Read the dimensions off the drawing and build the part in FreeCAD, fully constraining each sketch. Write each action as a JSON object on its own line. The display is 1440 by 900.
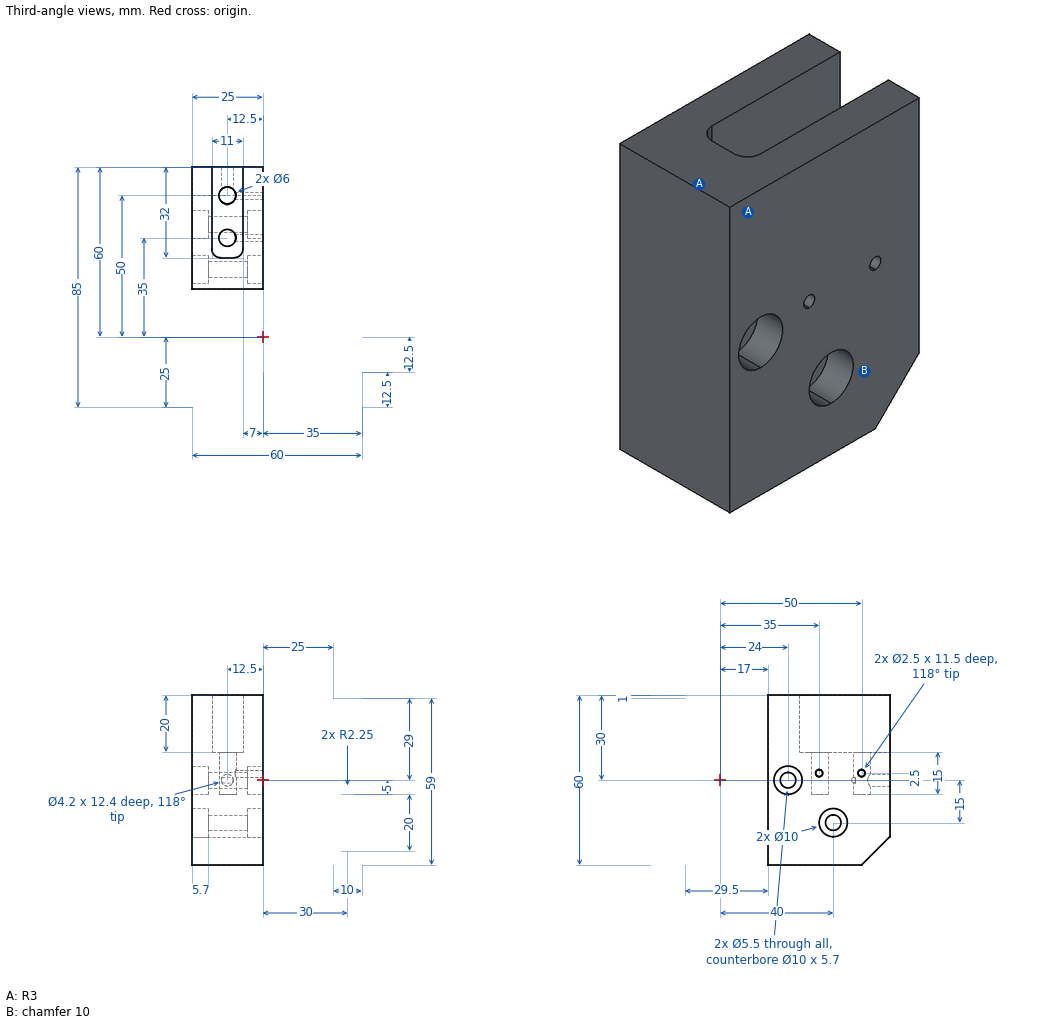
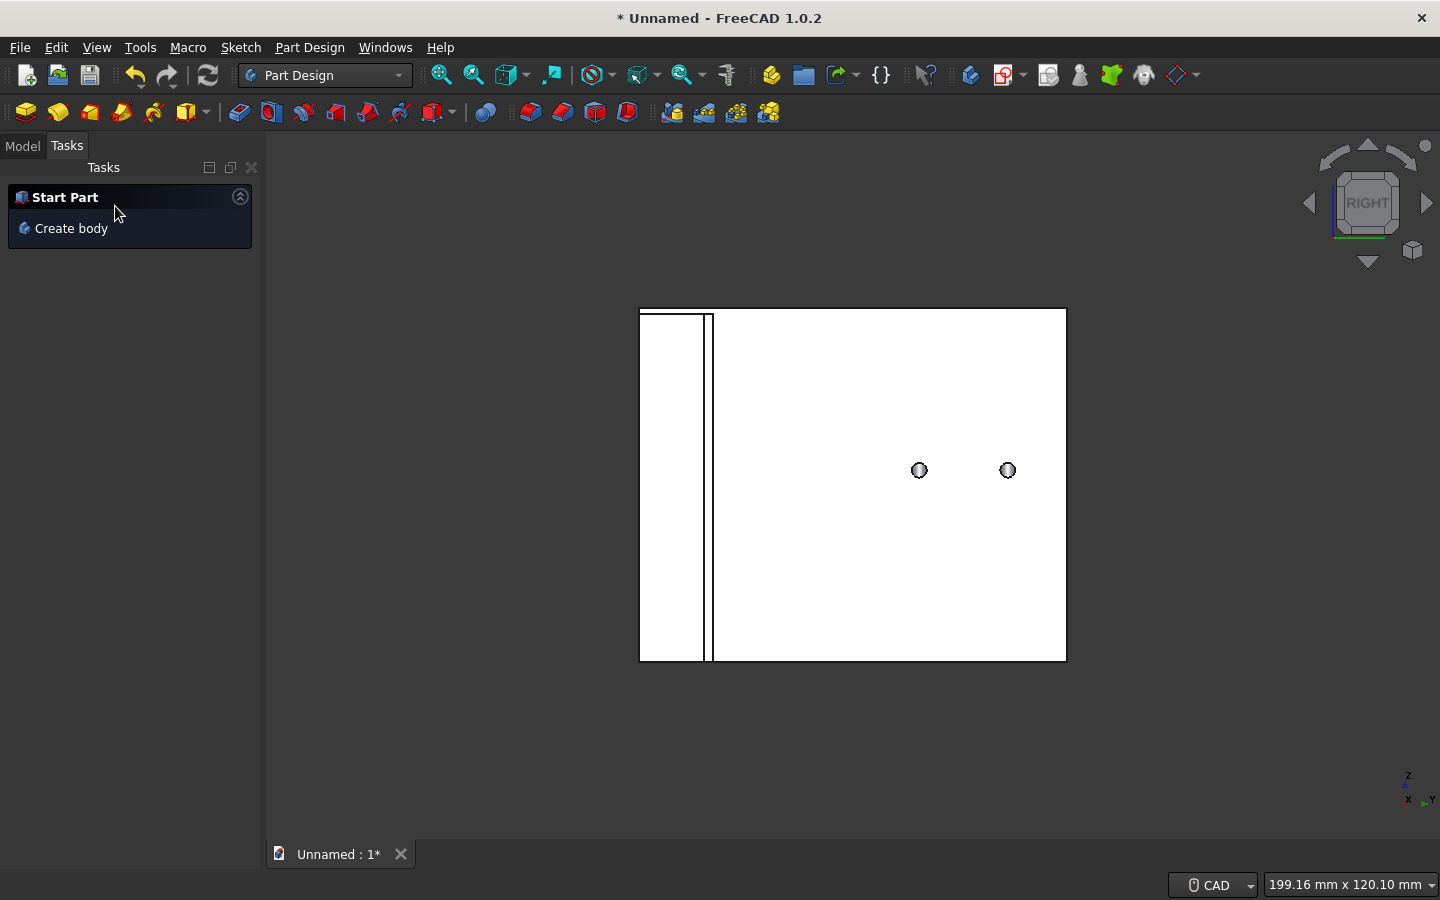
{"action": "key", "text": "5"}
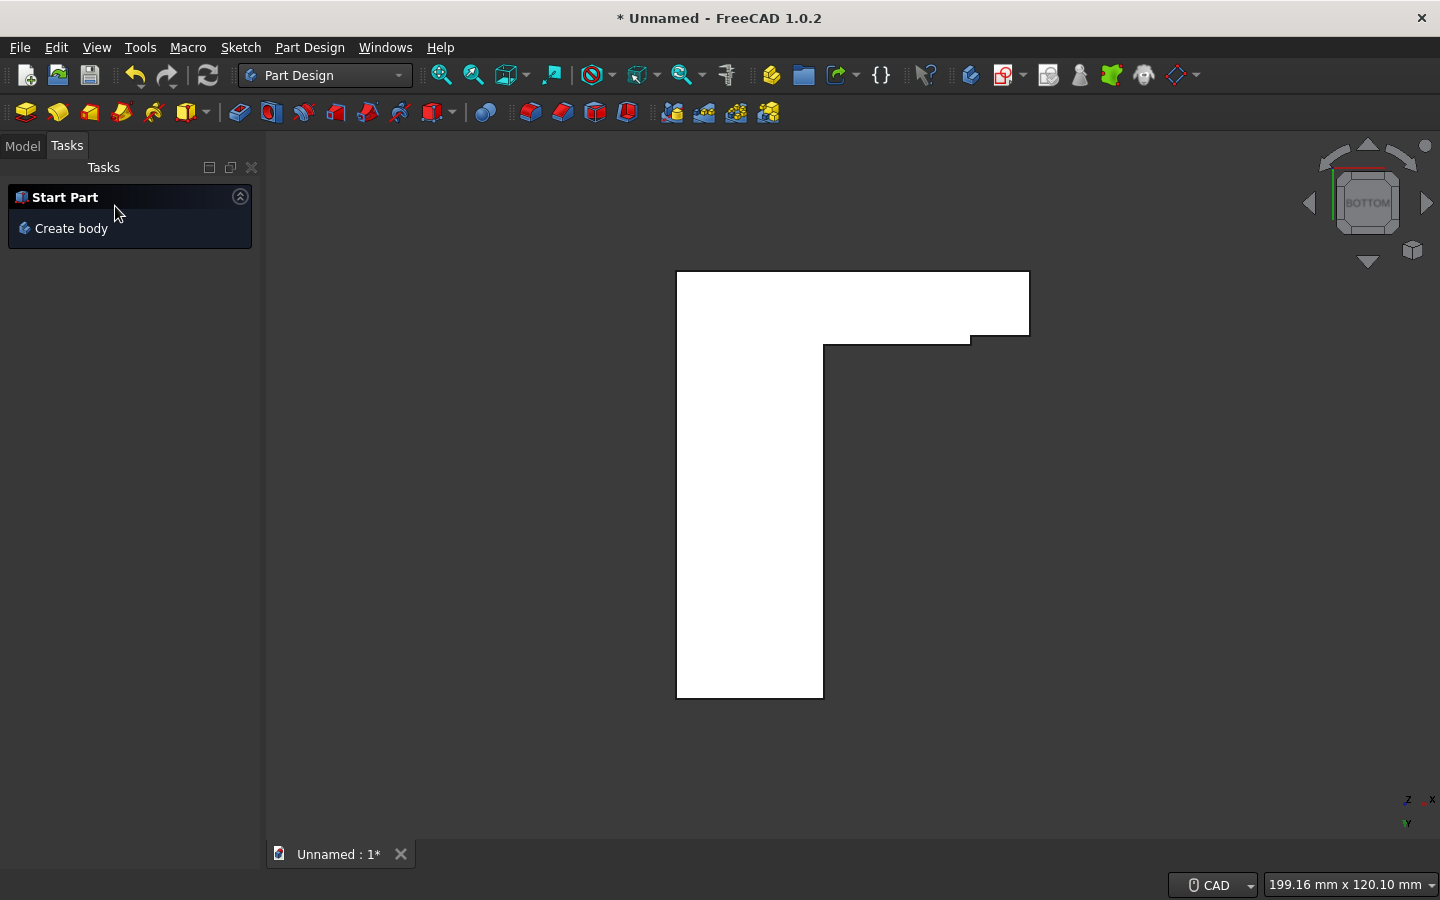
{"action": "left_click", "coordinate": [750, 698]}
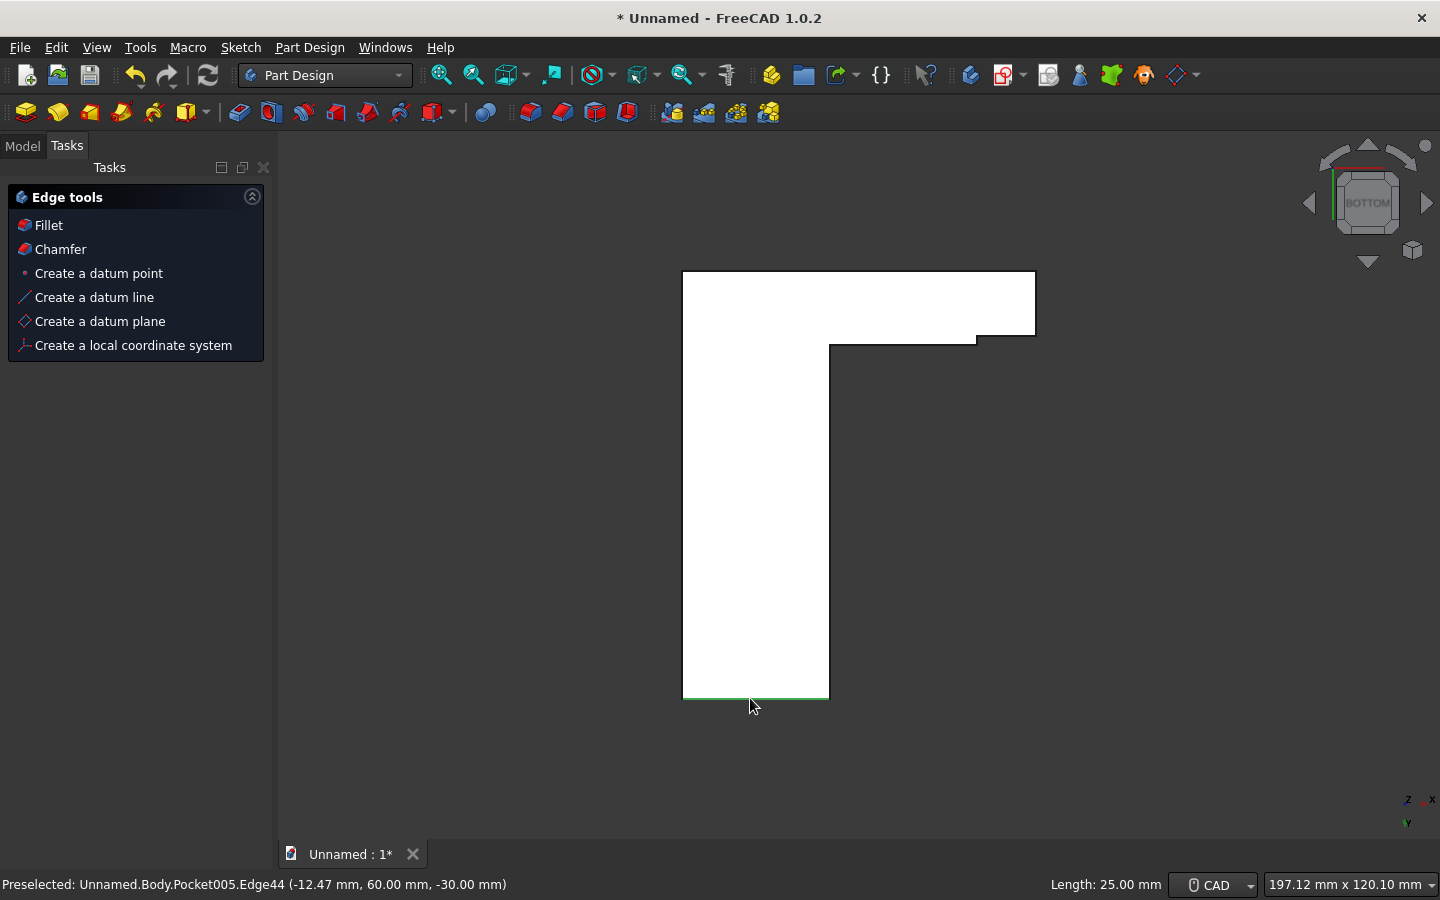
{"action": "left_click", "coordinate": [564, 112]}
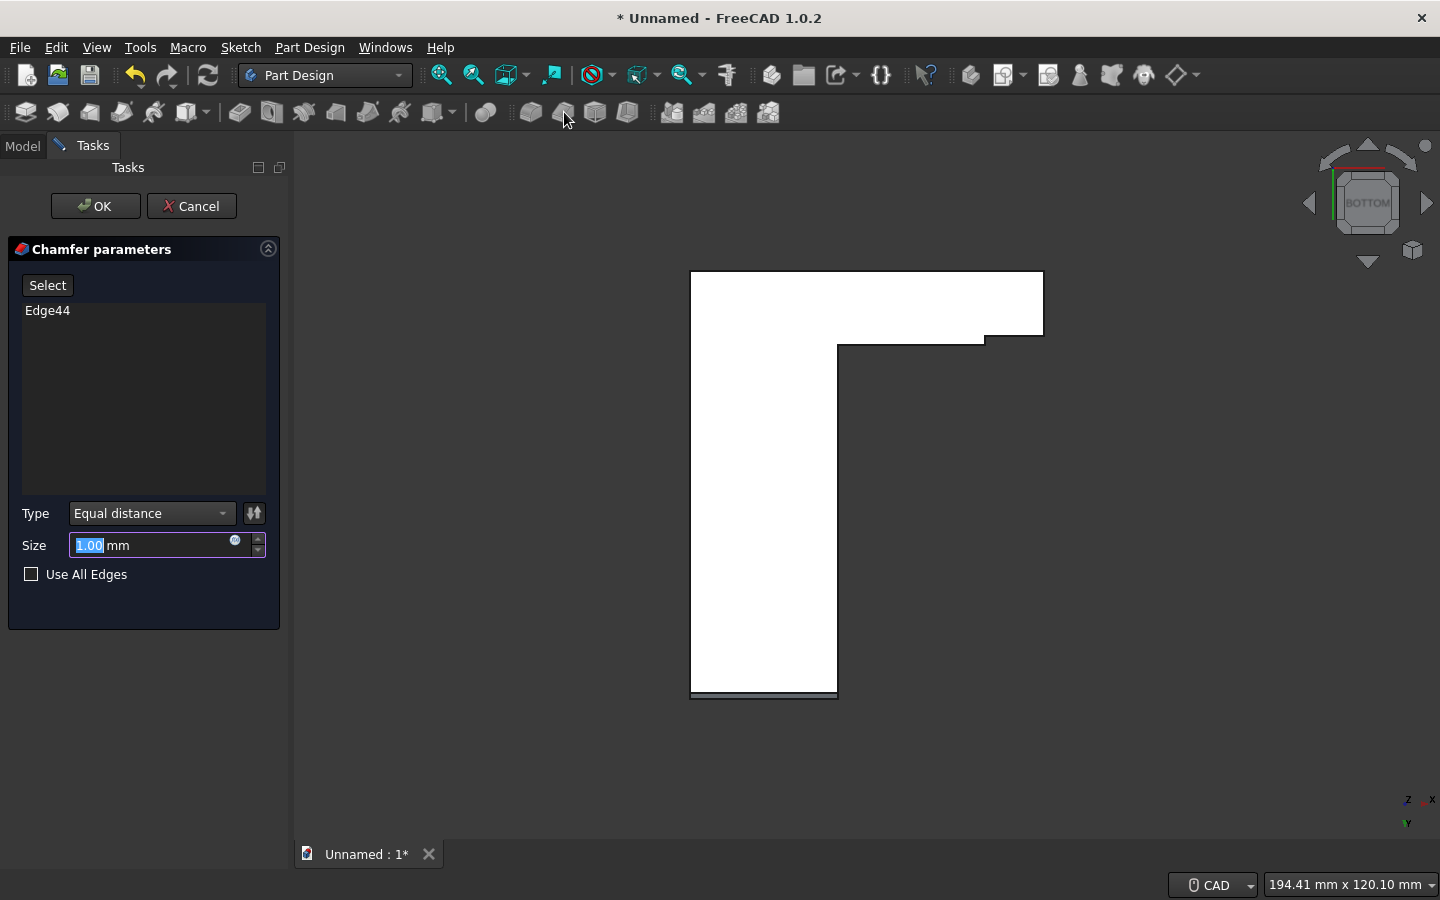
{"action": "type", "text": "10"}
{"action": "key", "text": "Tab"}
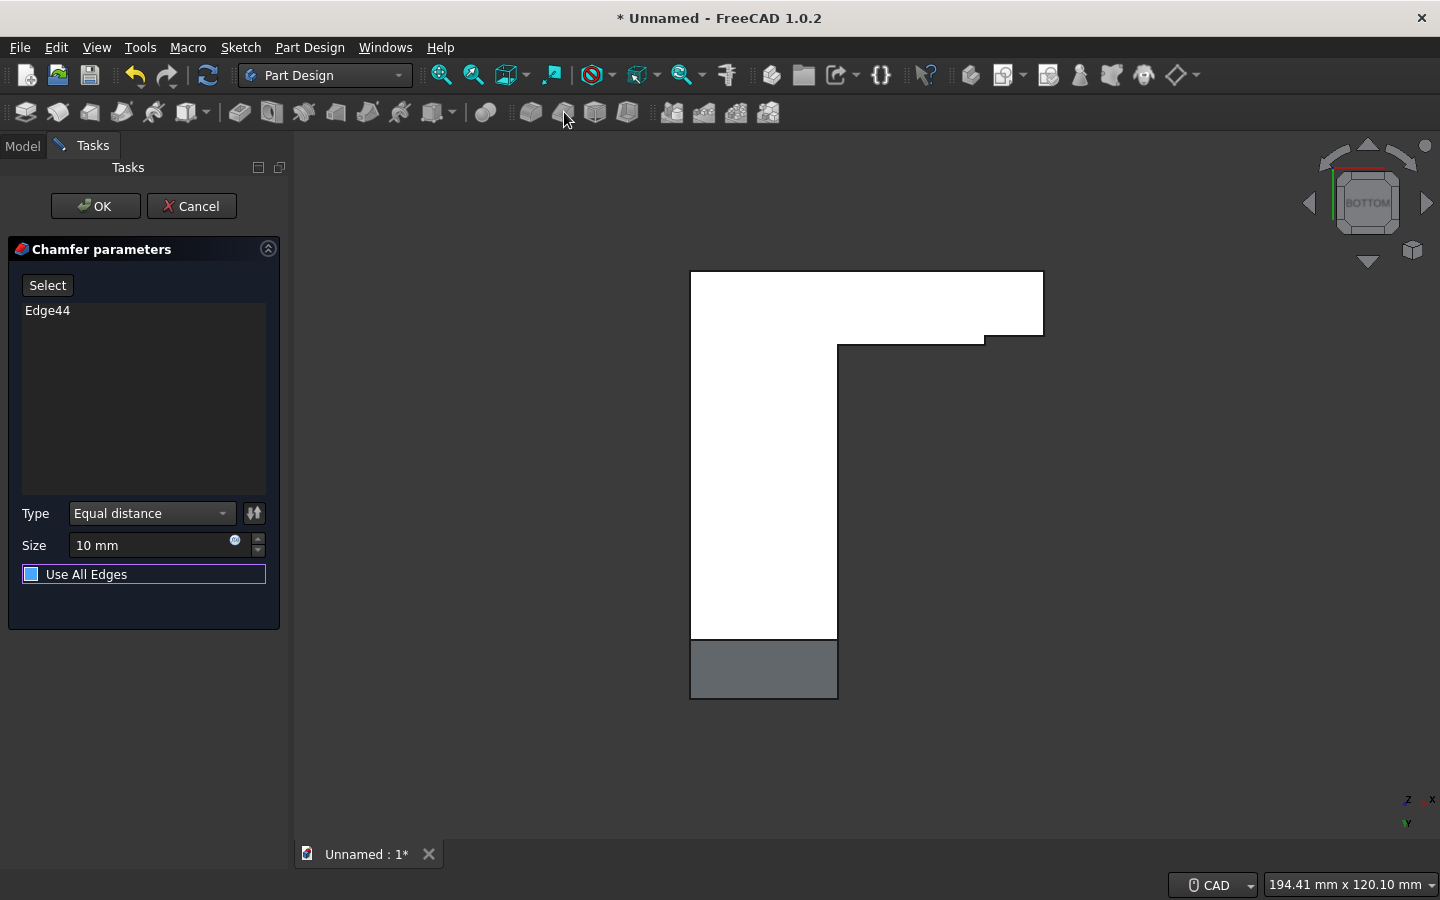
{"action": "left_click", "coordinate": [96, 206]}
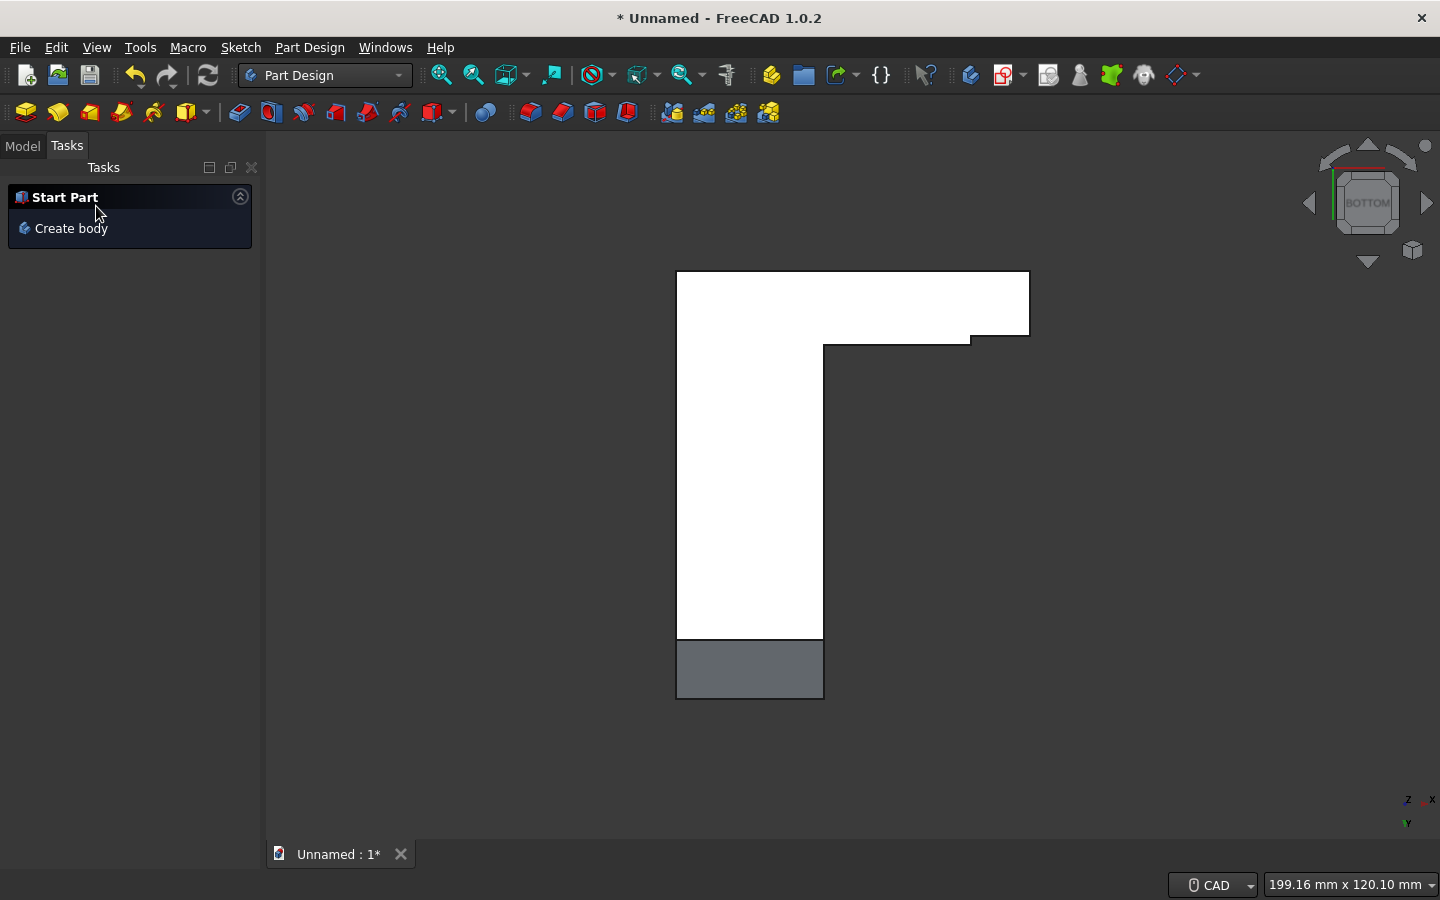
{"action": "key", "text": "0"}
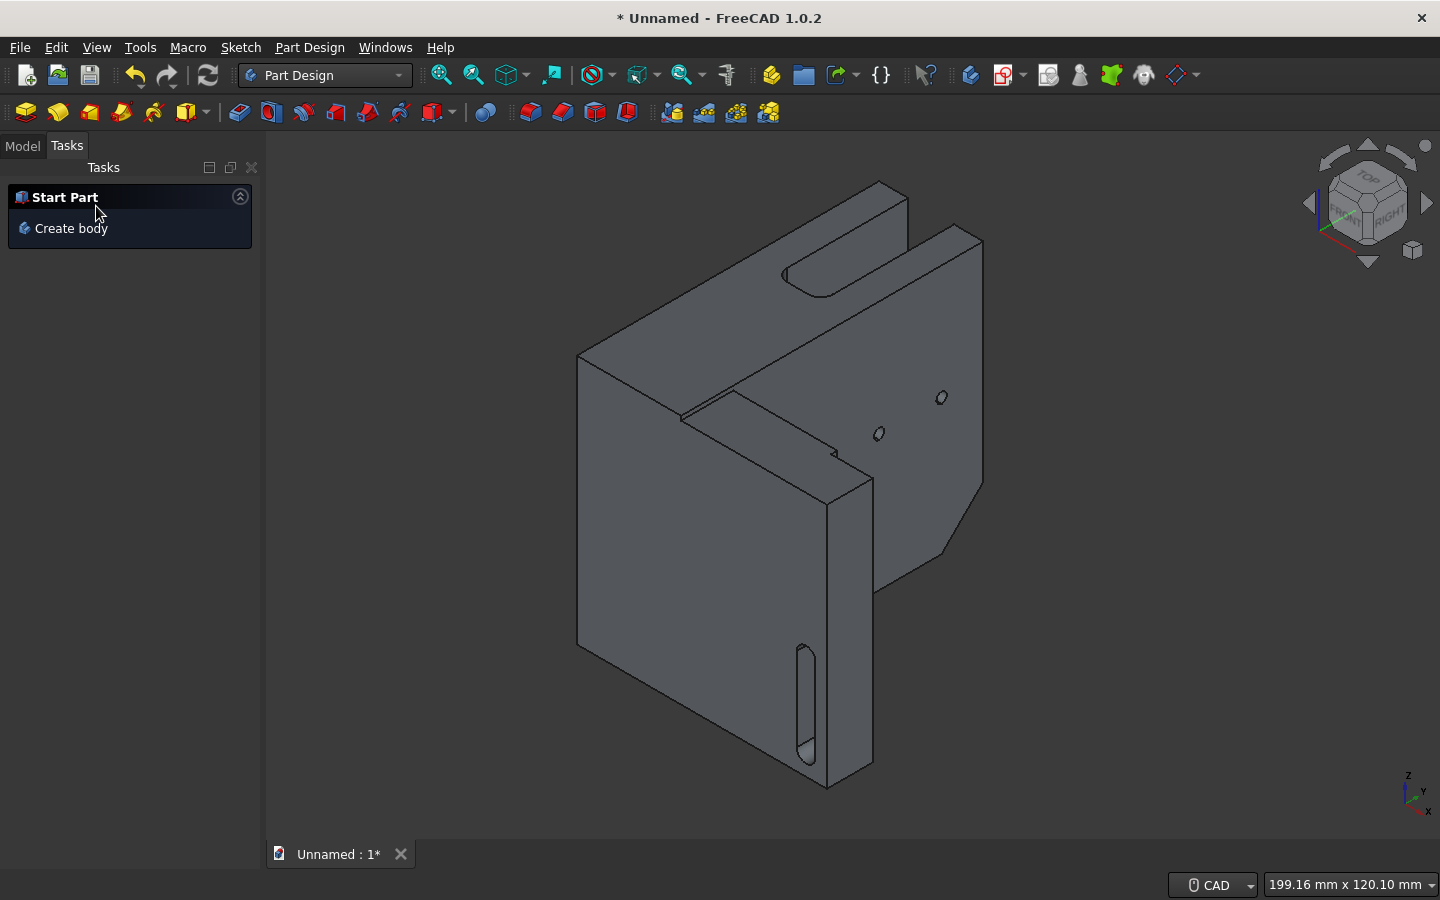
{"action": "left_click", "coordinate": [780, 447]}